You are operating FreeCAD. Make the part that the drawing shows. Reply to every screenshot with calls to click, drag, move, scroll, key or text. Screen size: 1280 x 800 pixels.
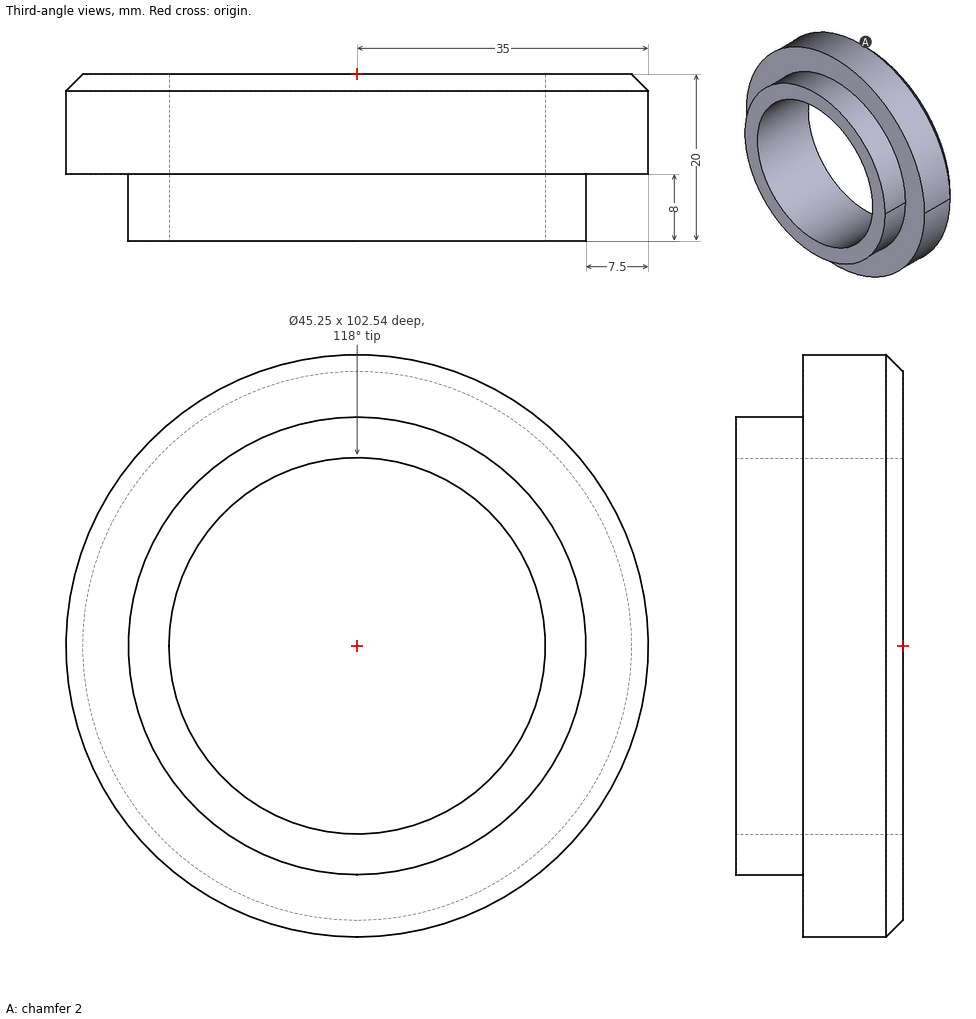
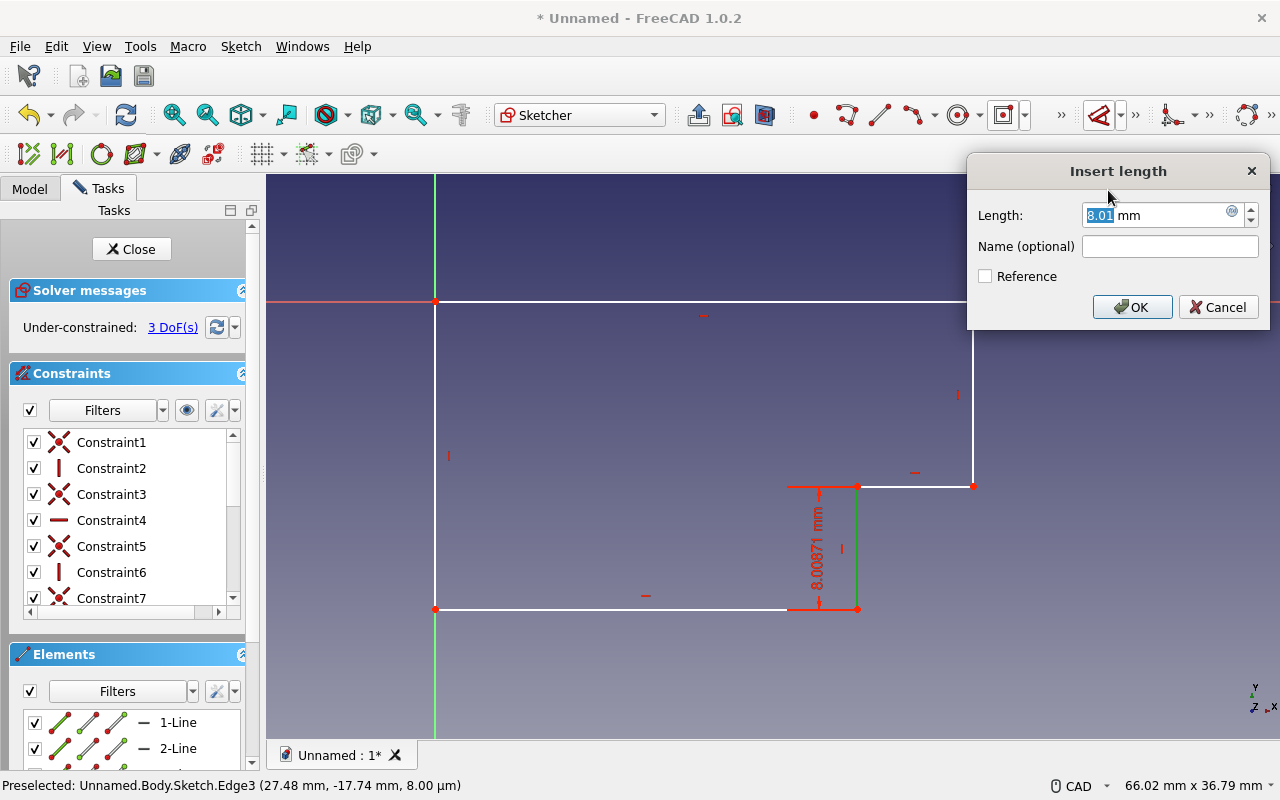
text(8)
key(Return)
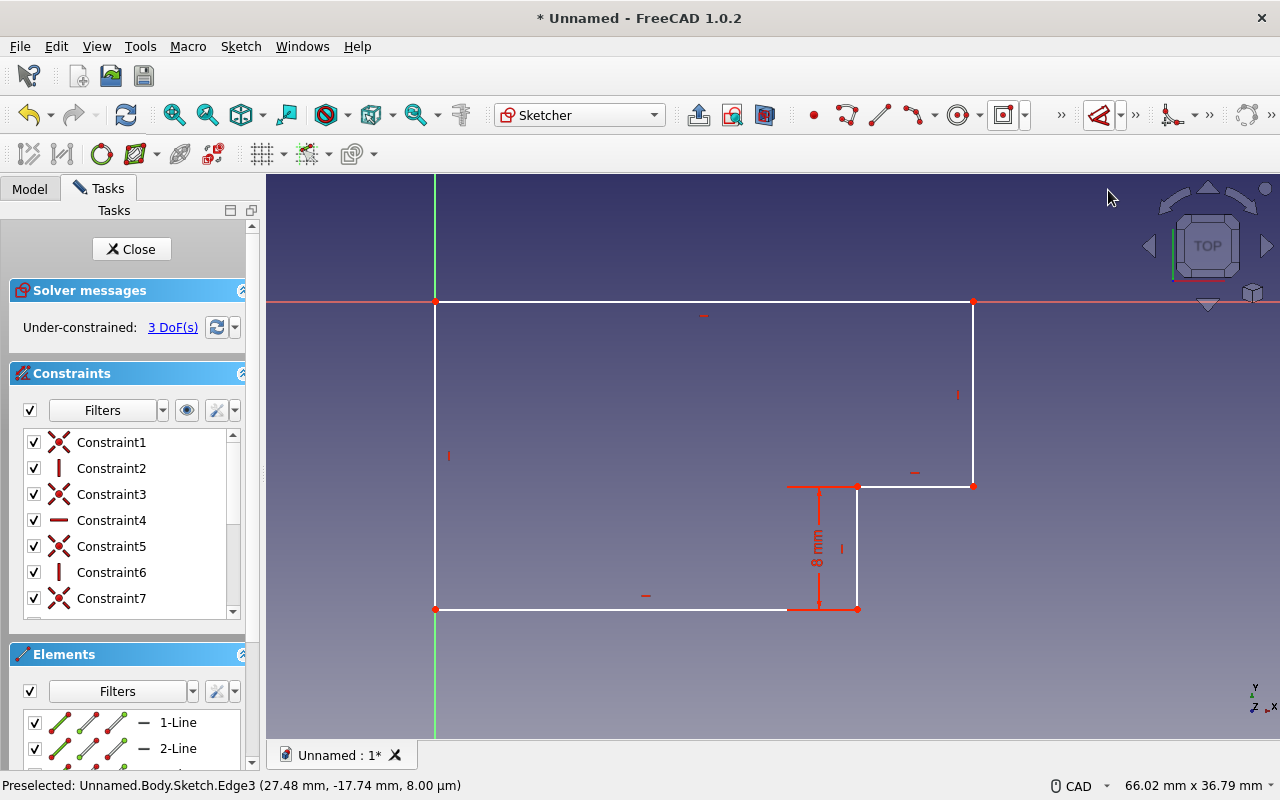
click(435, 394)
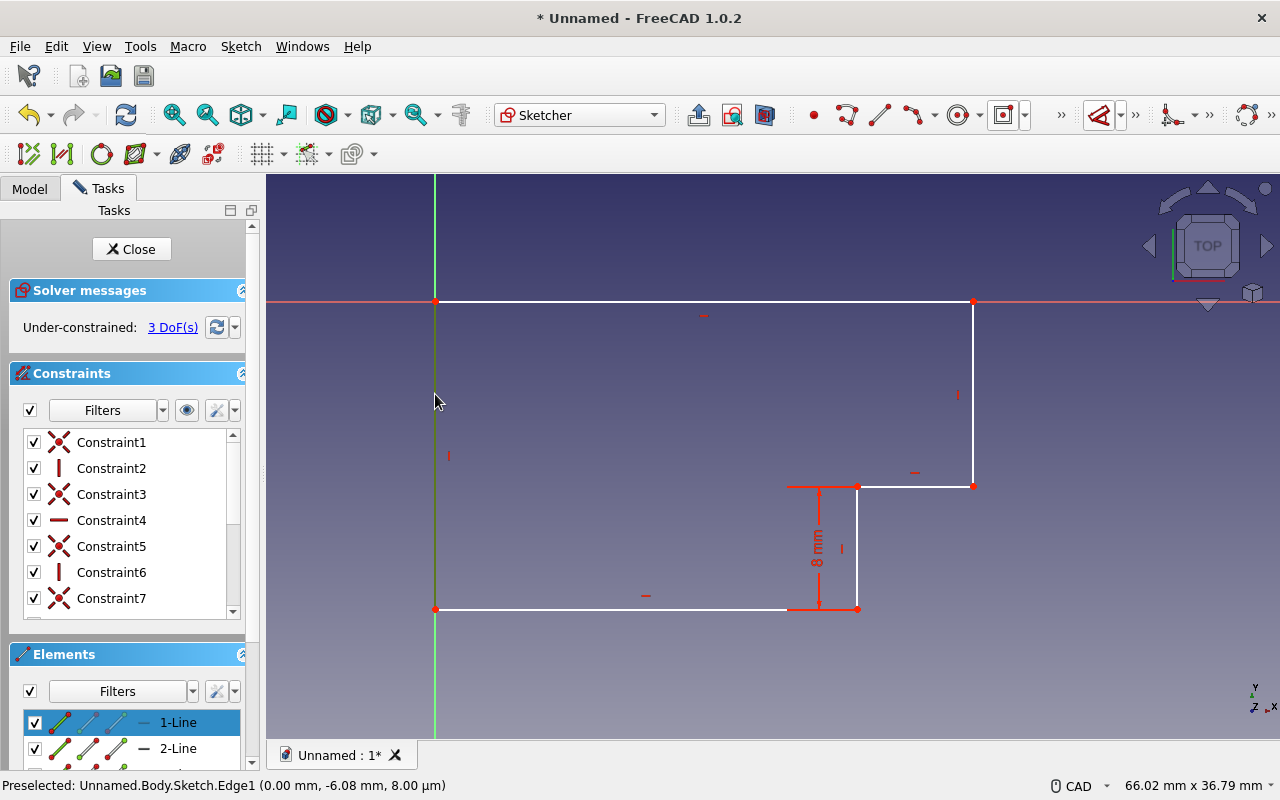
click(1120, 116)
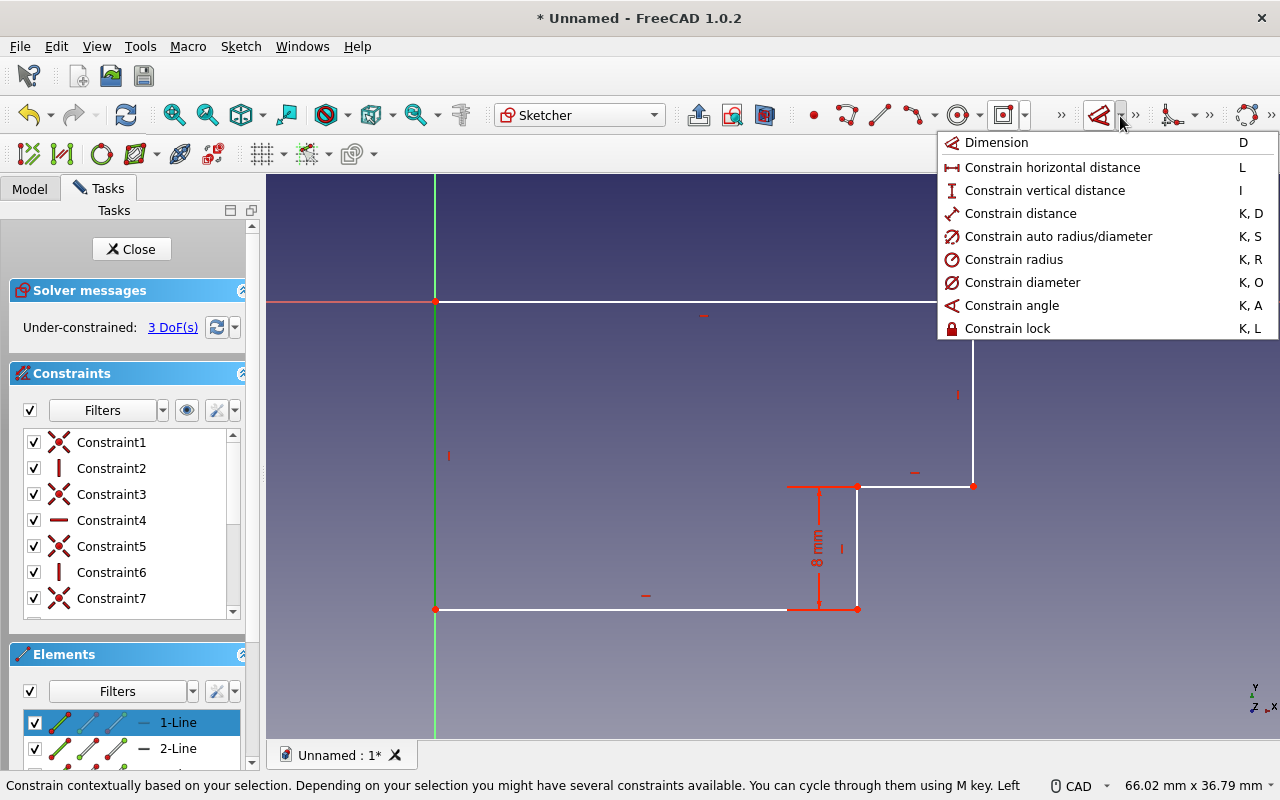
click(1108, 190)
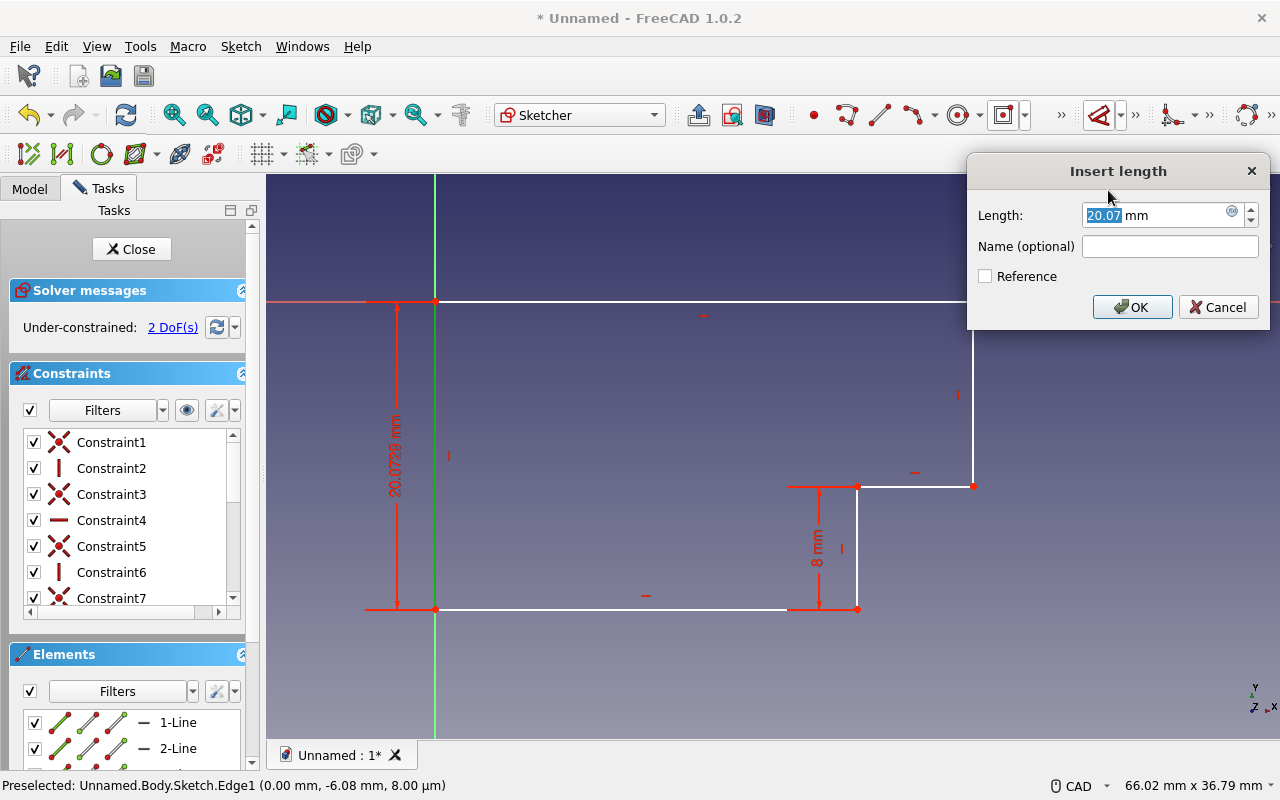
text(20)
key(Return)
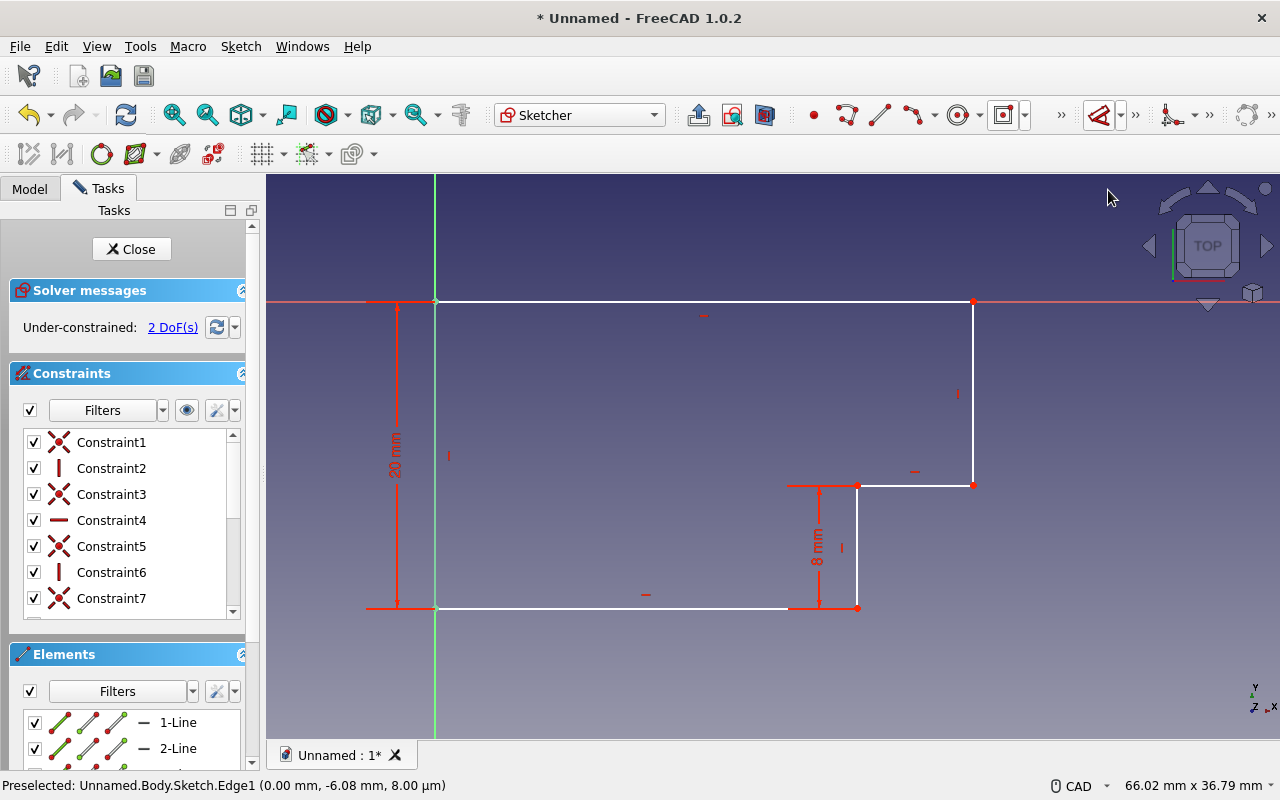
click(812, 302)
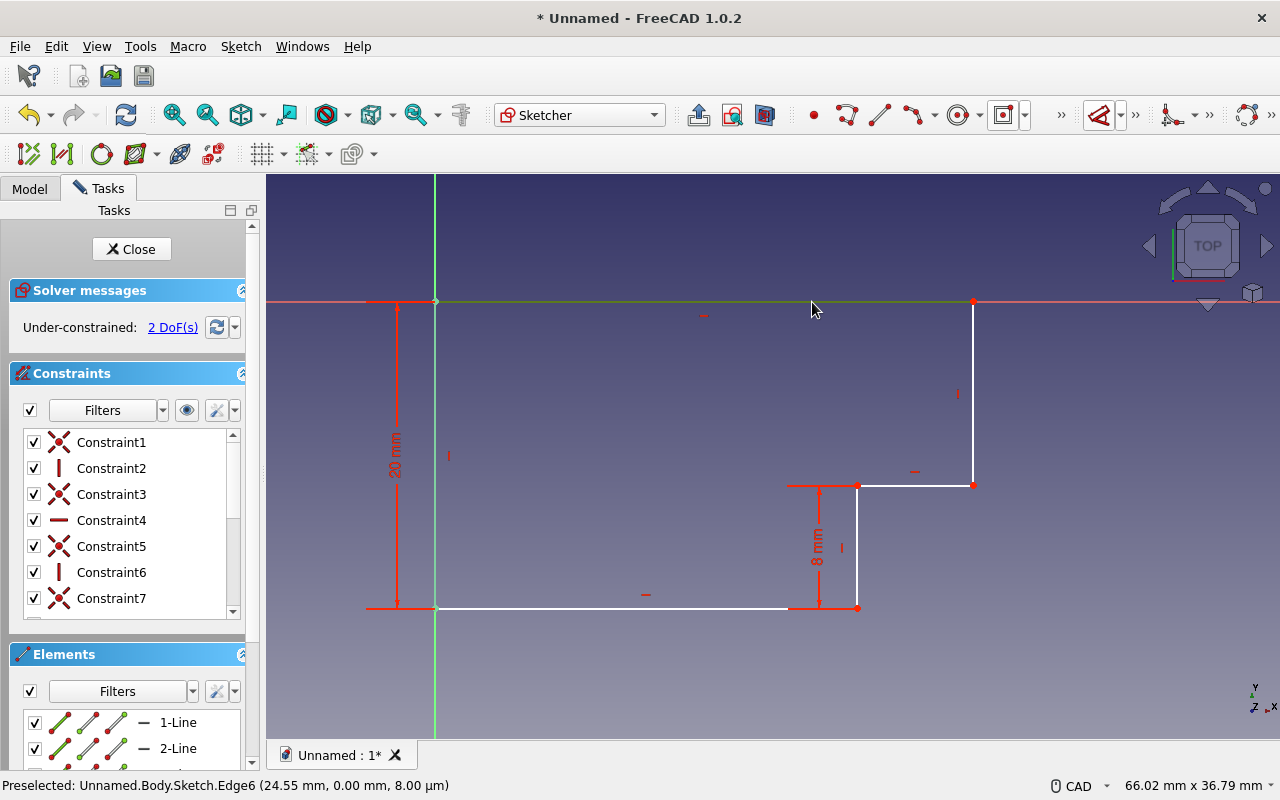
key(l)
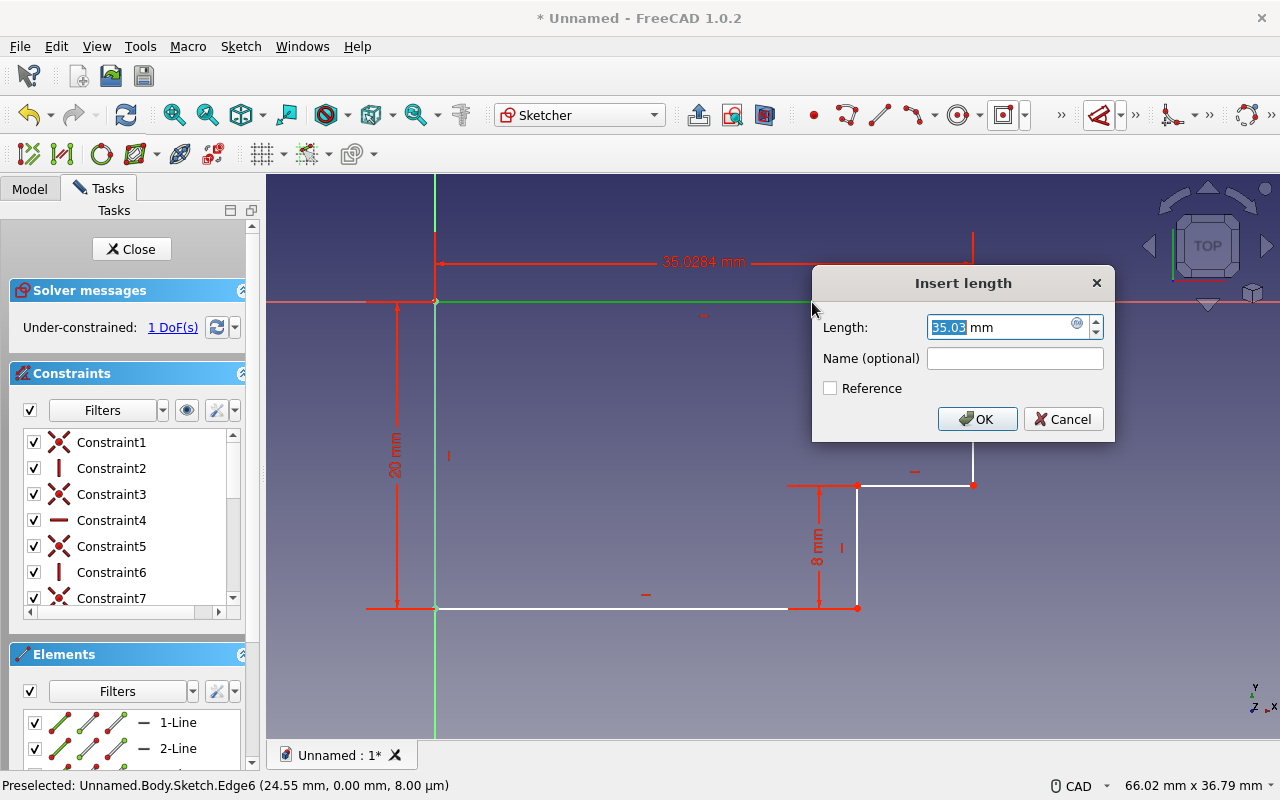
text(35)
key(Return)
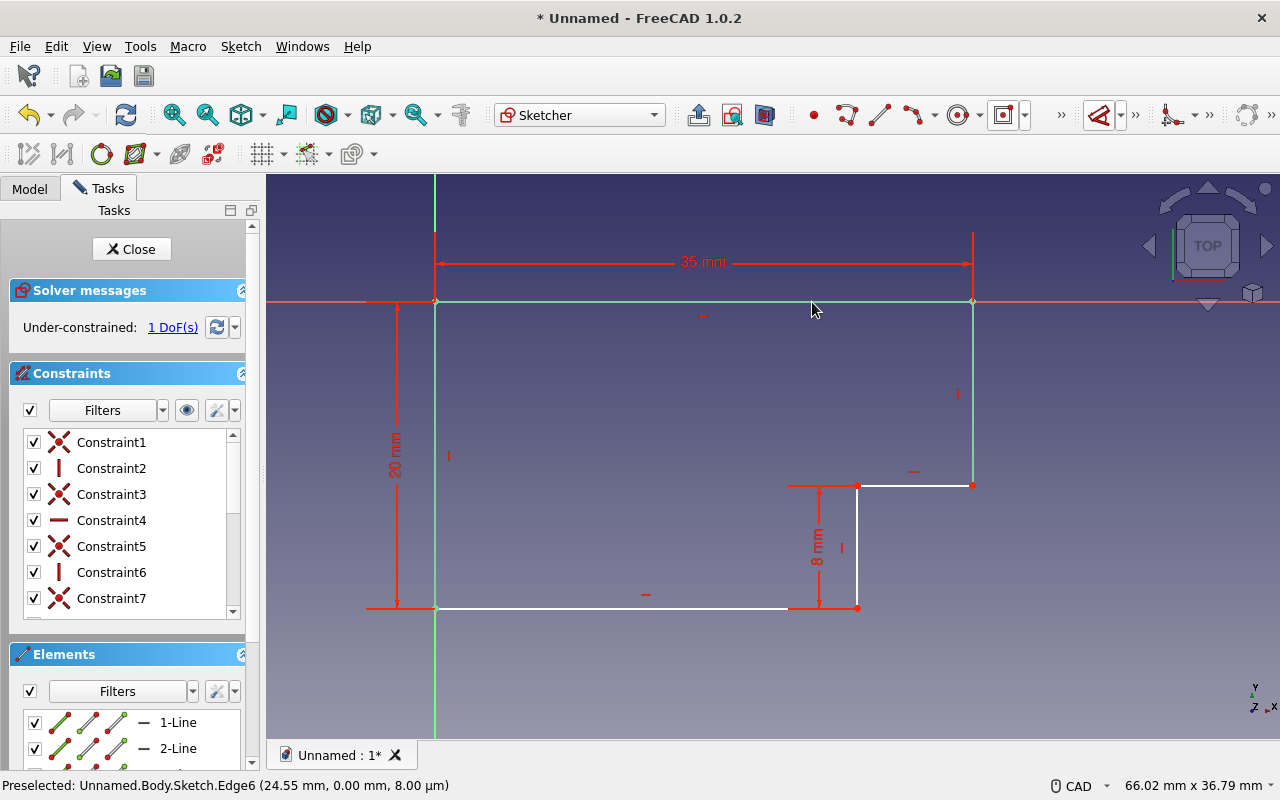
click(892, 486)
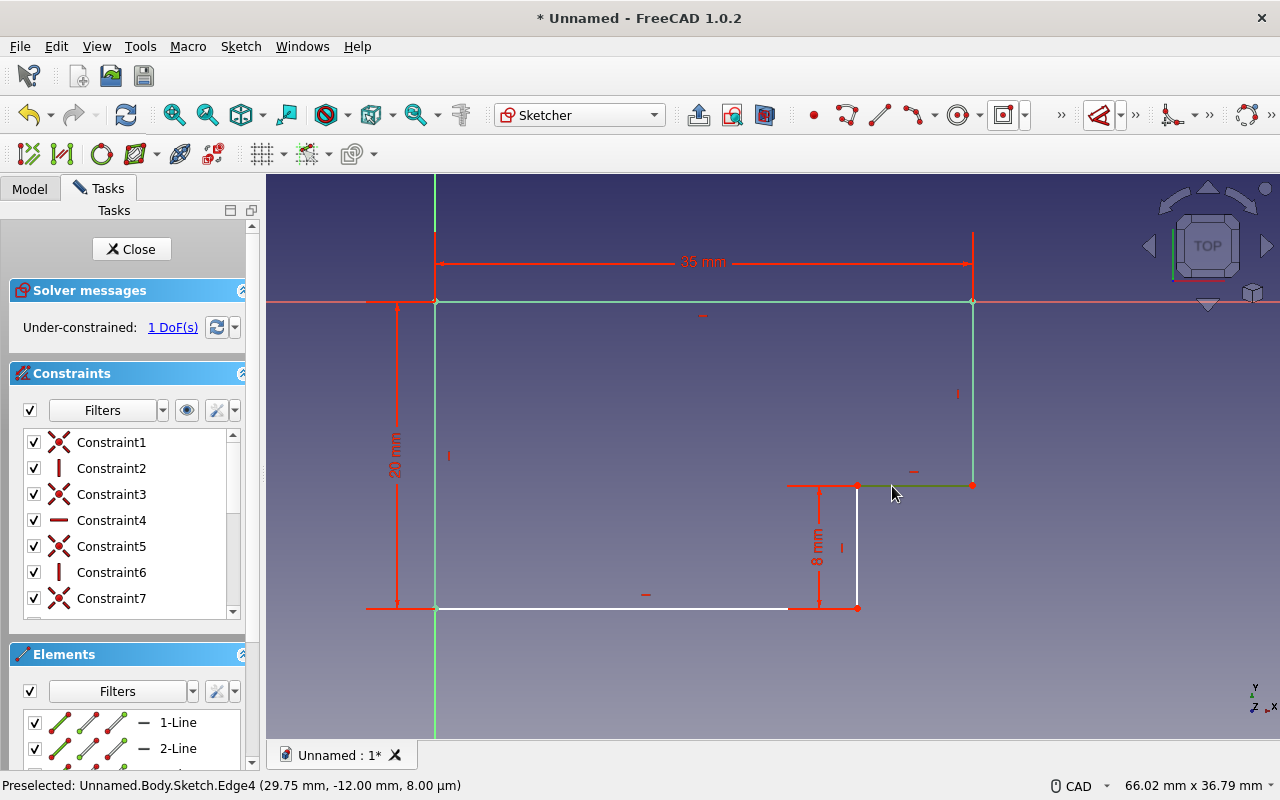
click(1120, 116)